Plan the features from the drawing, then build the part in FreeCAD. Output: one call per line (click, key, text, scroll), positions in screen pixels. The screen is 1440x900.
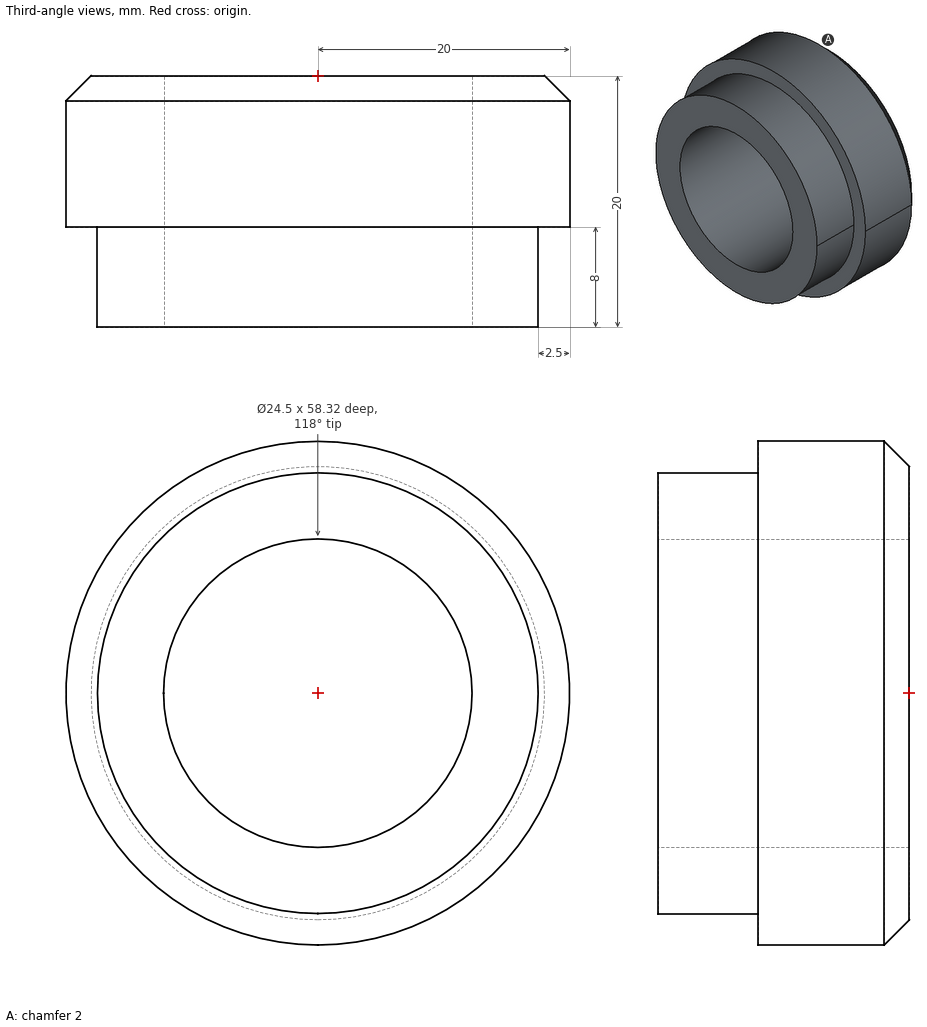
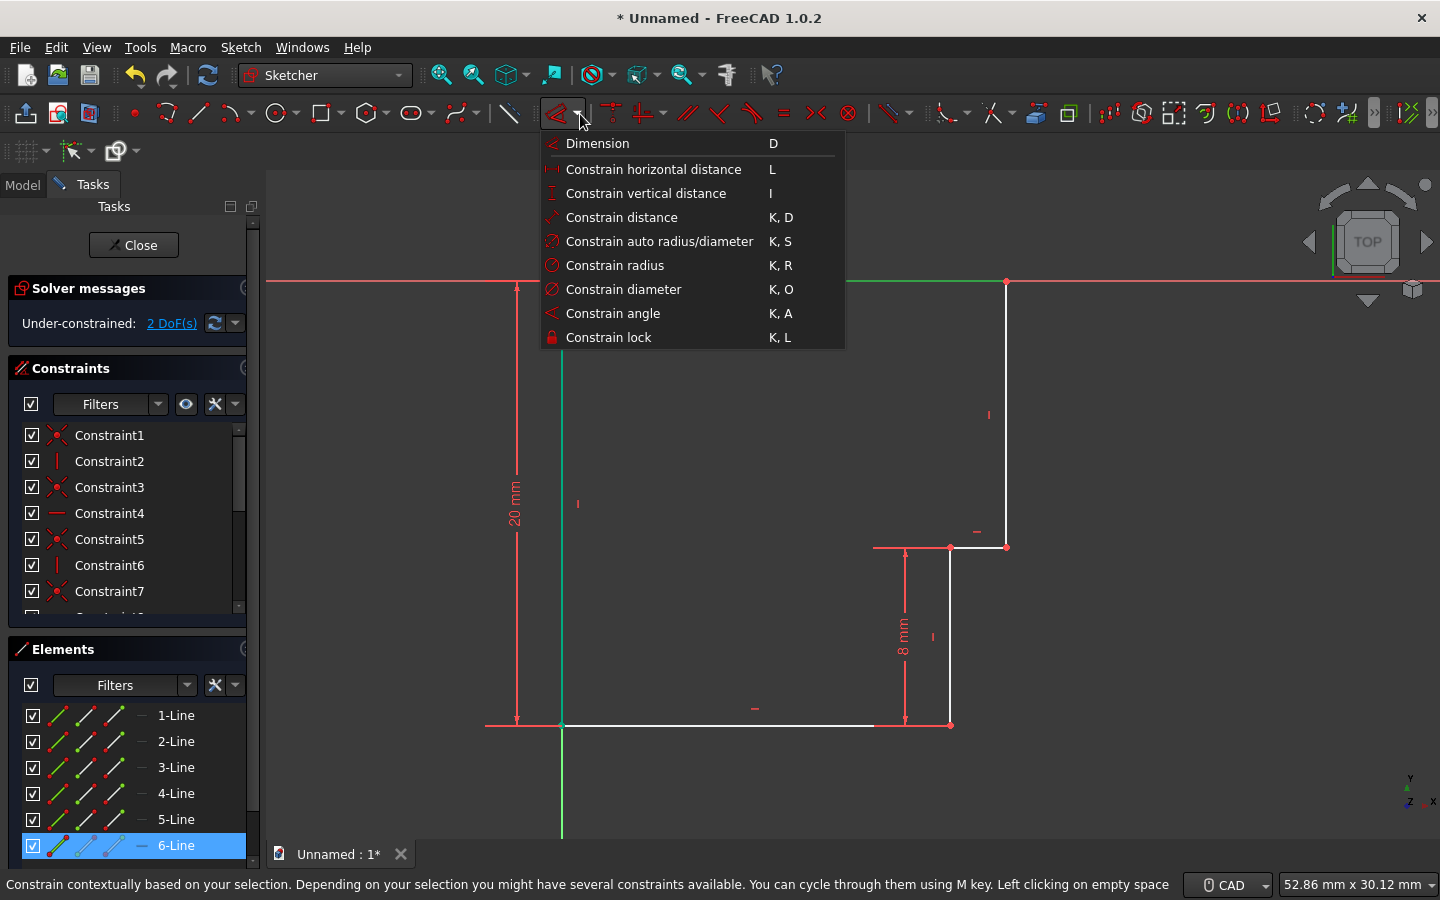
click(693, 169)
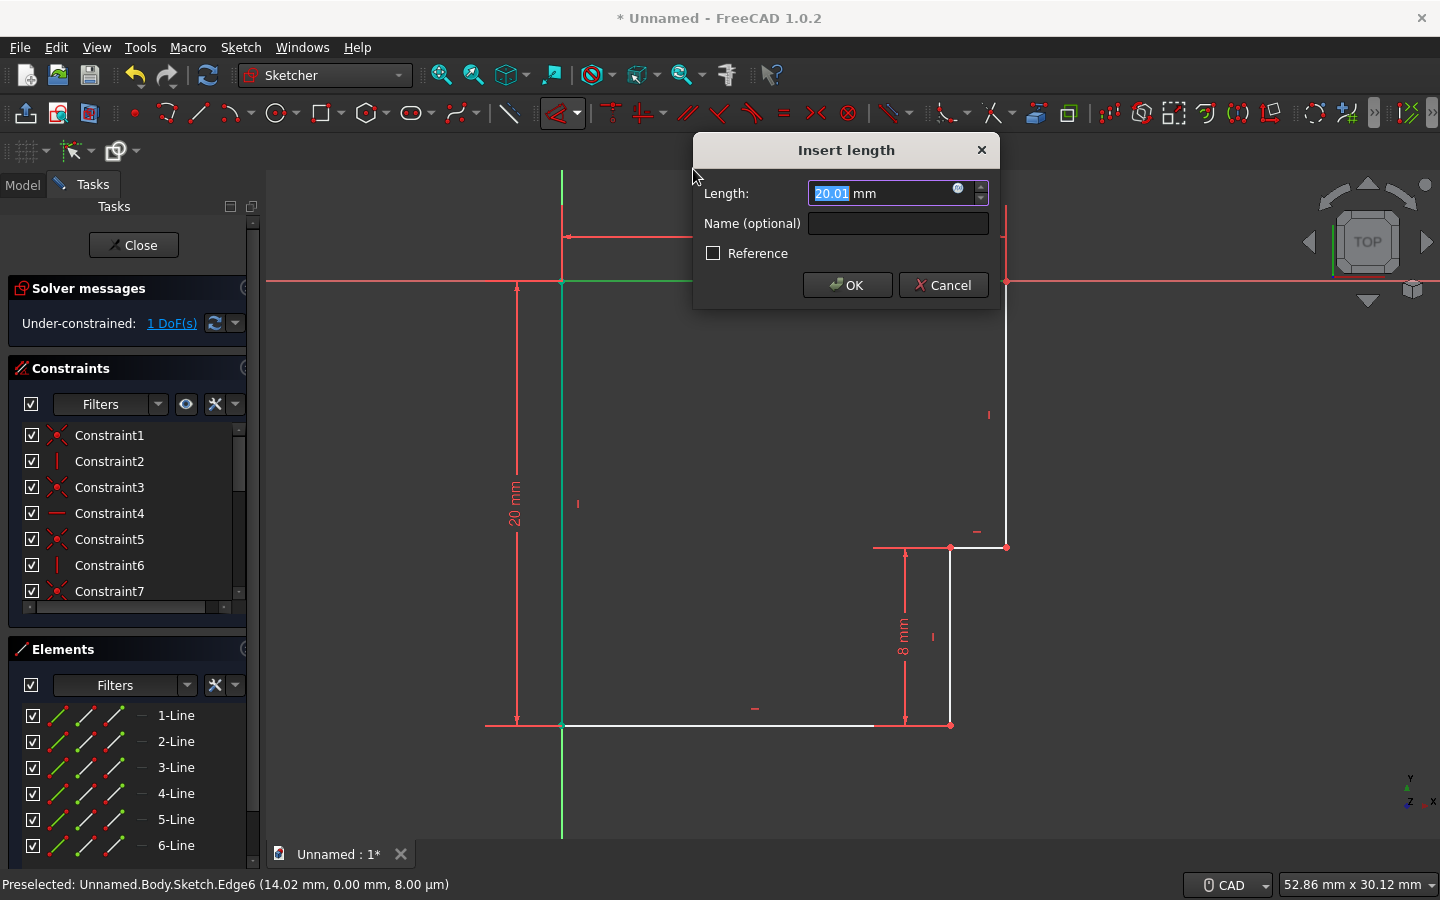
text(20)
key(Return)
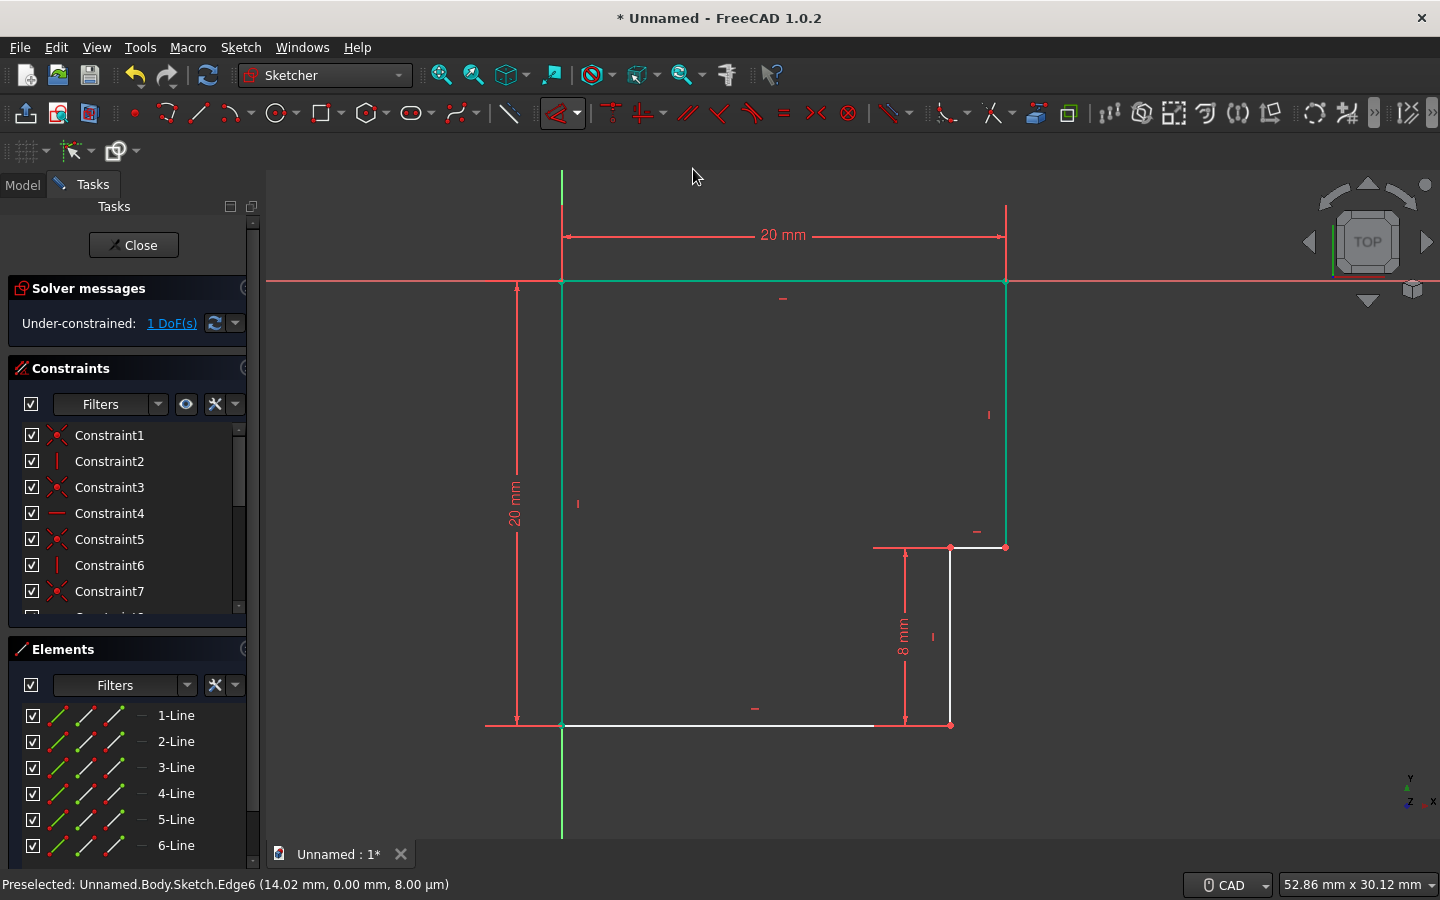
click(967, 548)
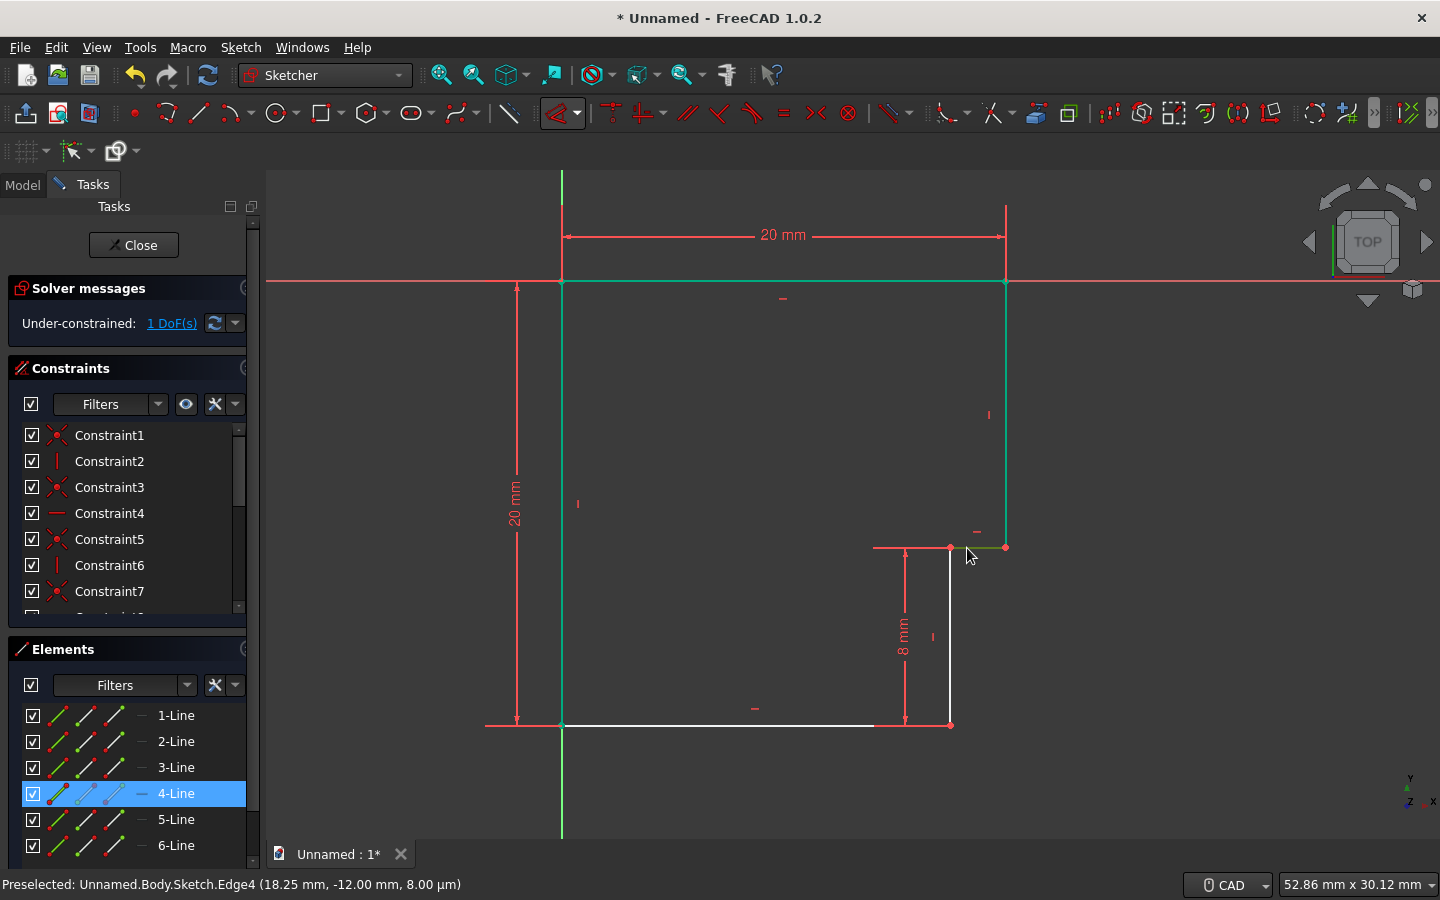
key(l)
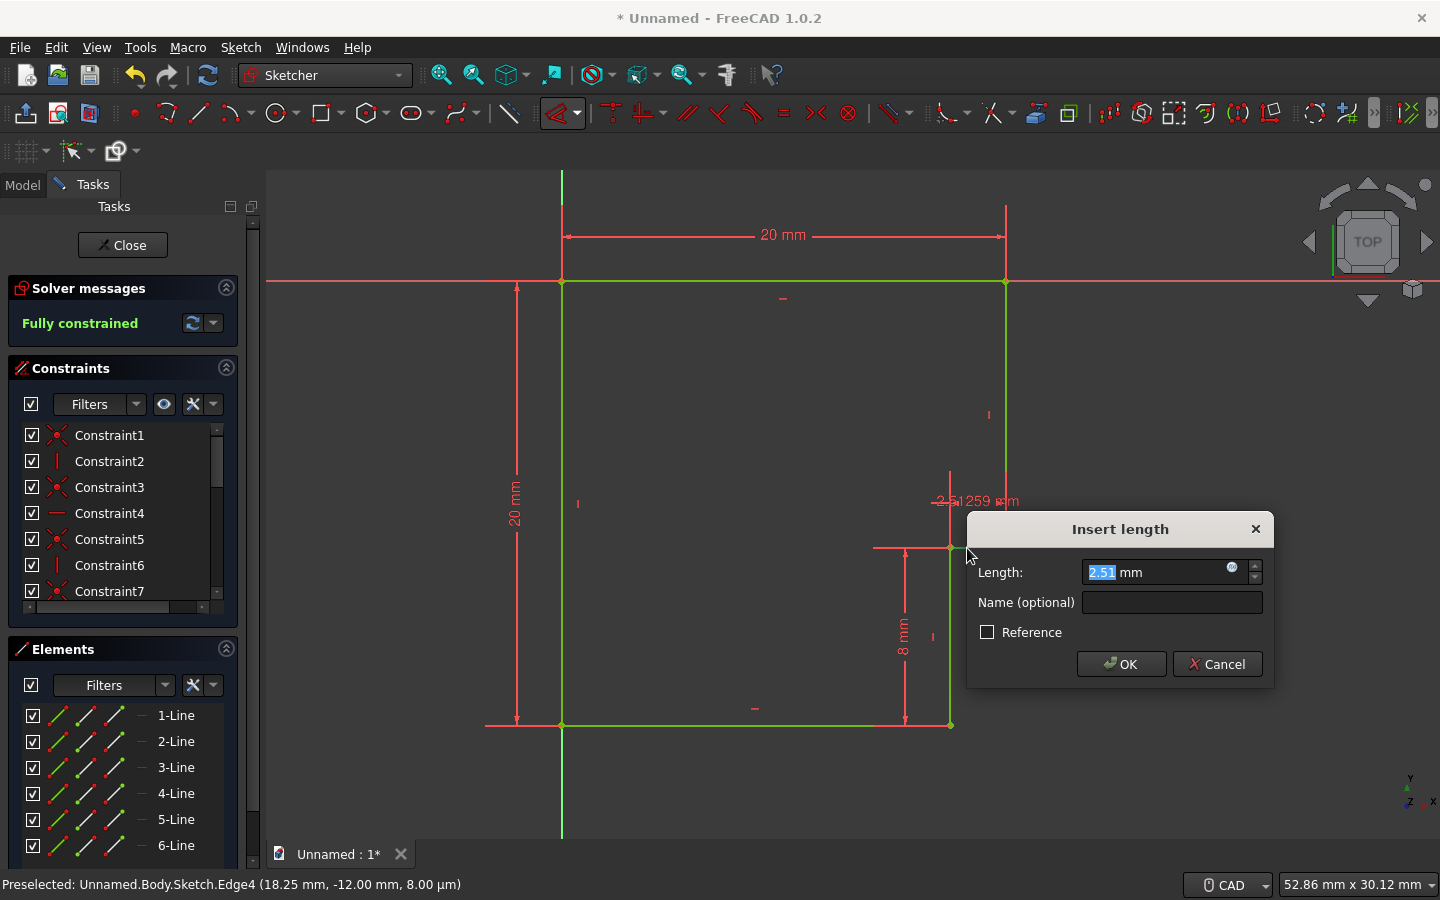
text(2.5)
key(Return)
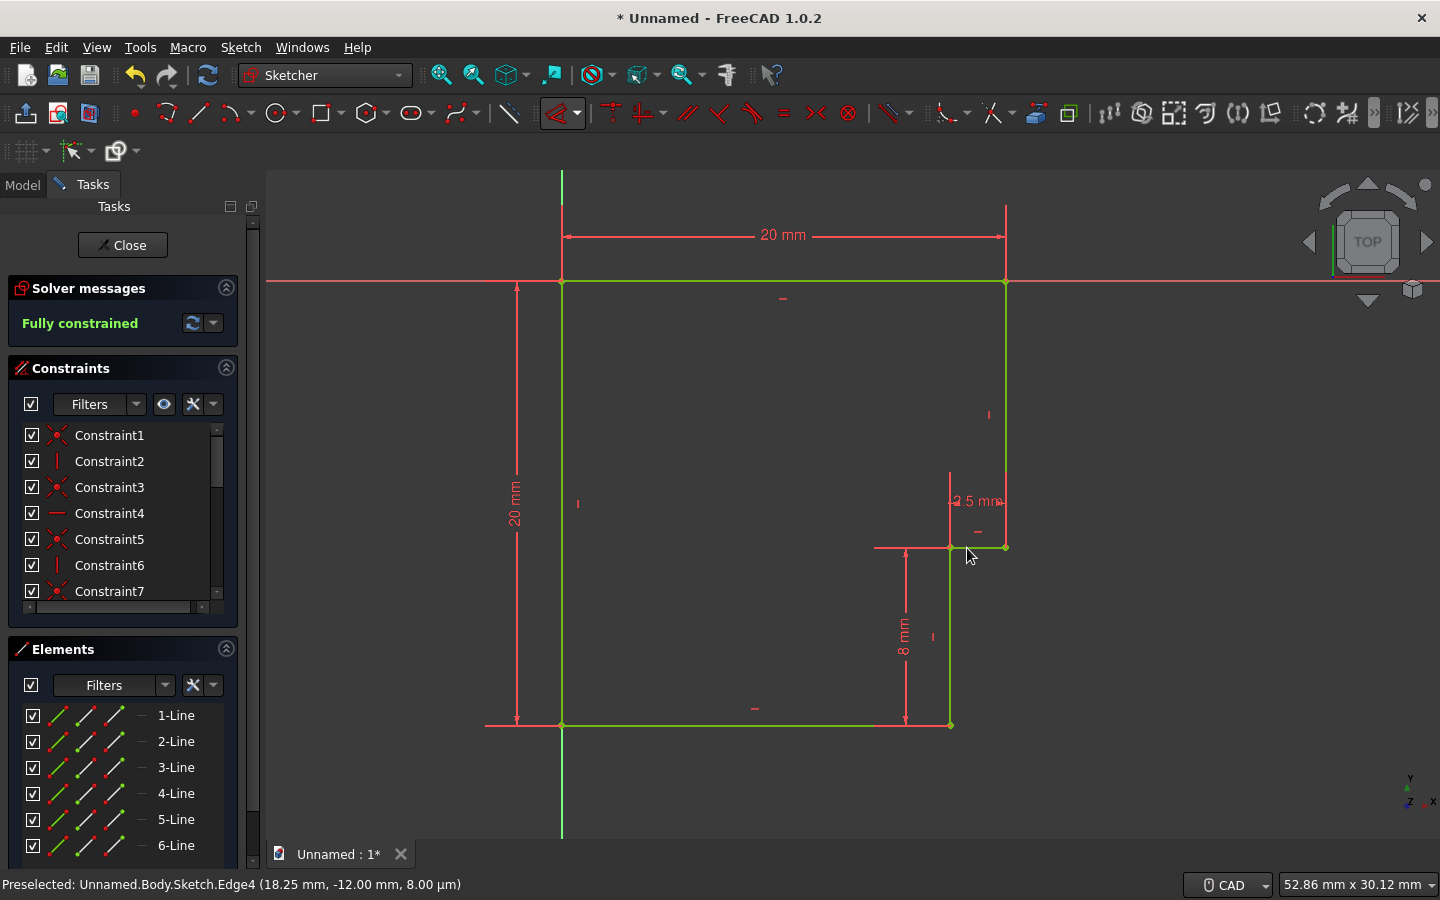
click(123, 245)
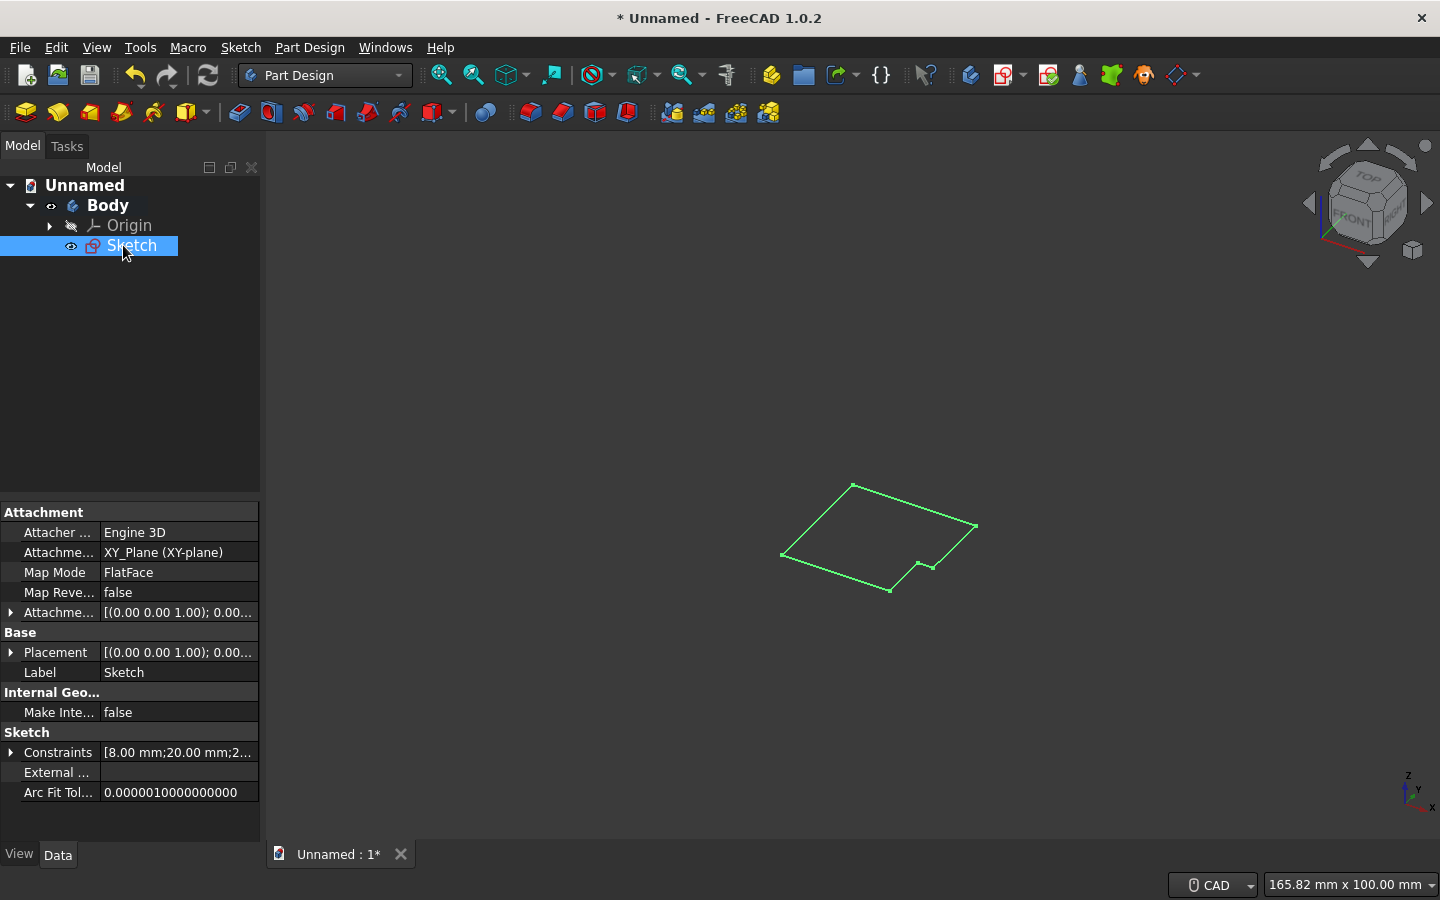
click(58, 112)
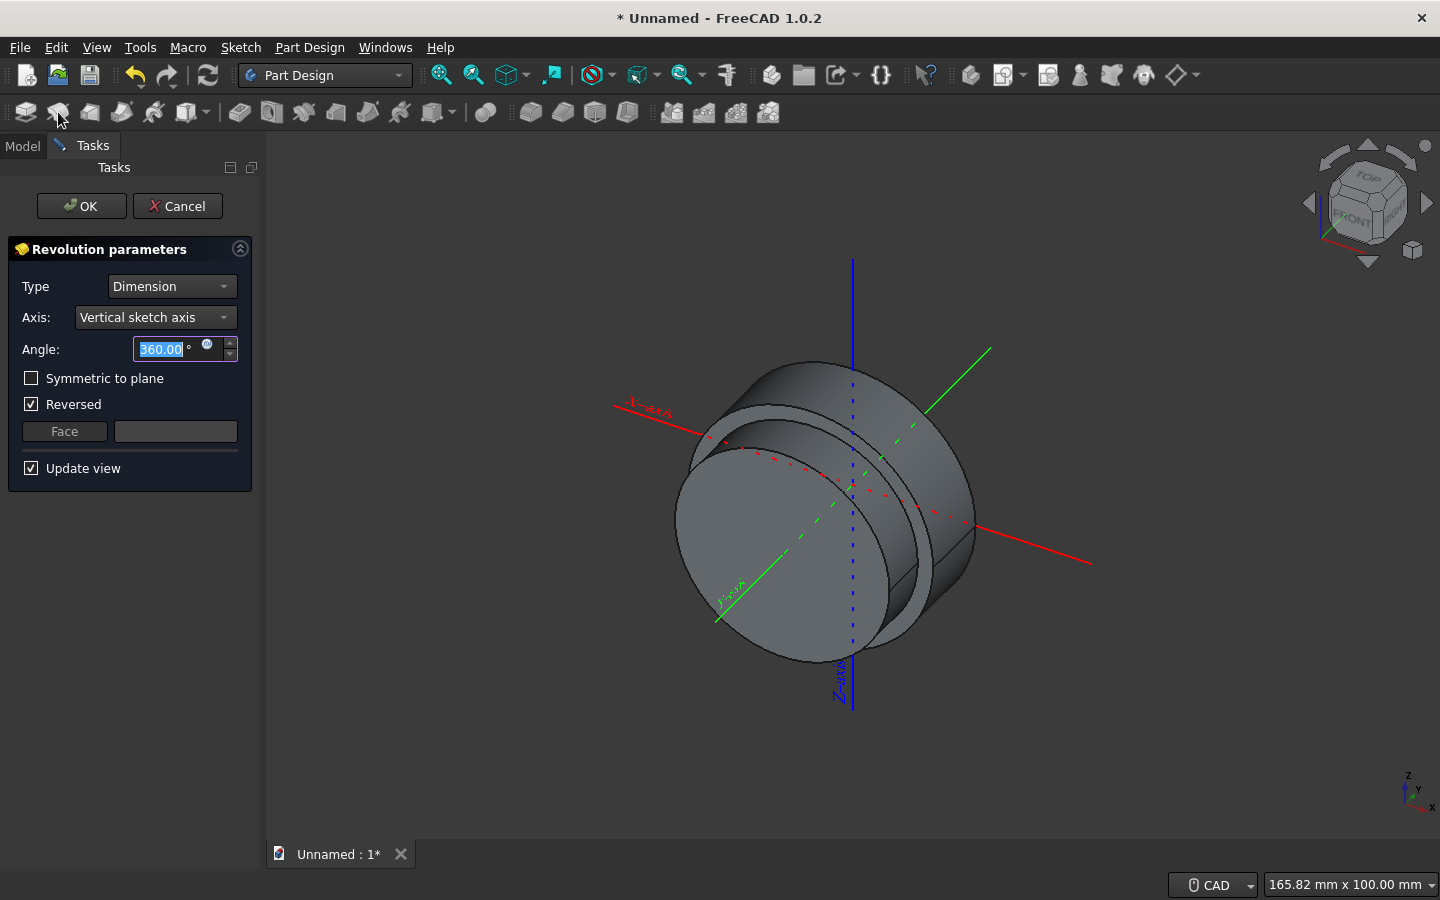
click(82, 206)